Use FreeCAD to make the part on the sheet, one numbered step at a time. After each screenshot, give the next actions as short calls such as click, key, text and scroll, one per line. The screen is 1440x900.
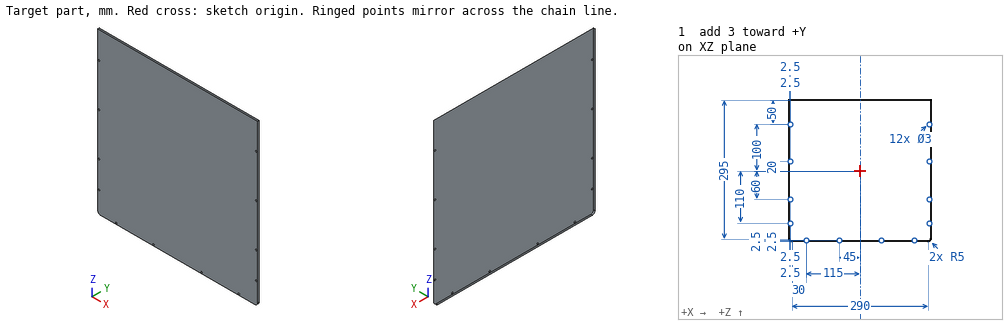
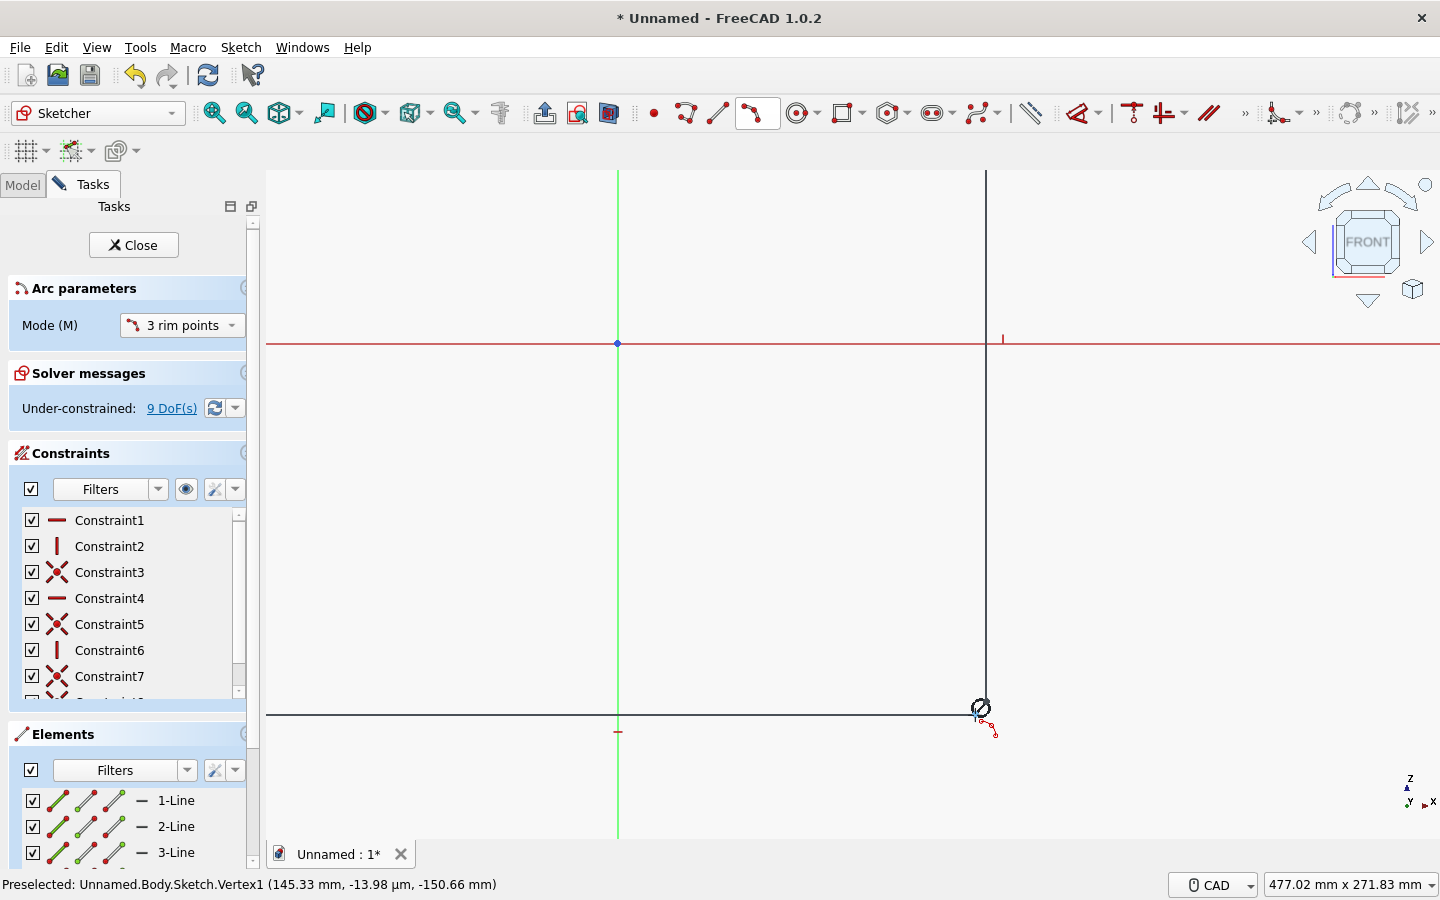
scroll(983, 709, up, 8)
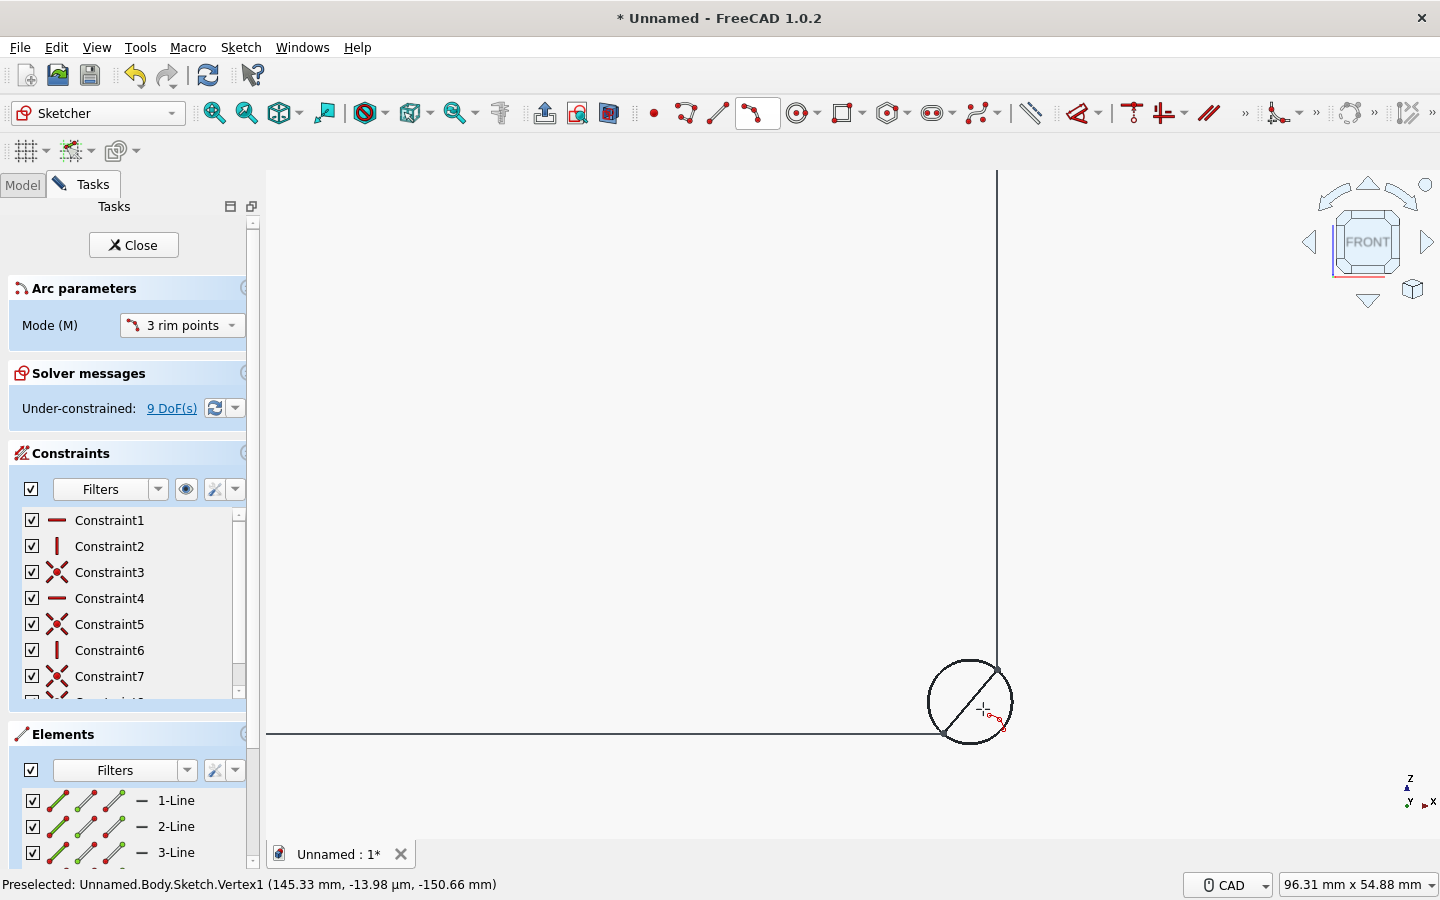
click(982, 708)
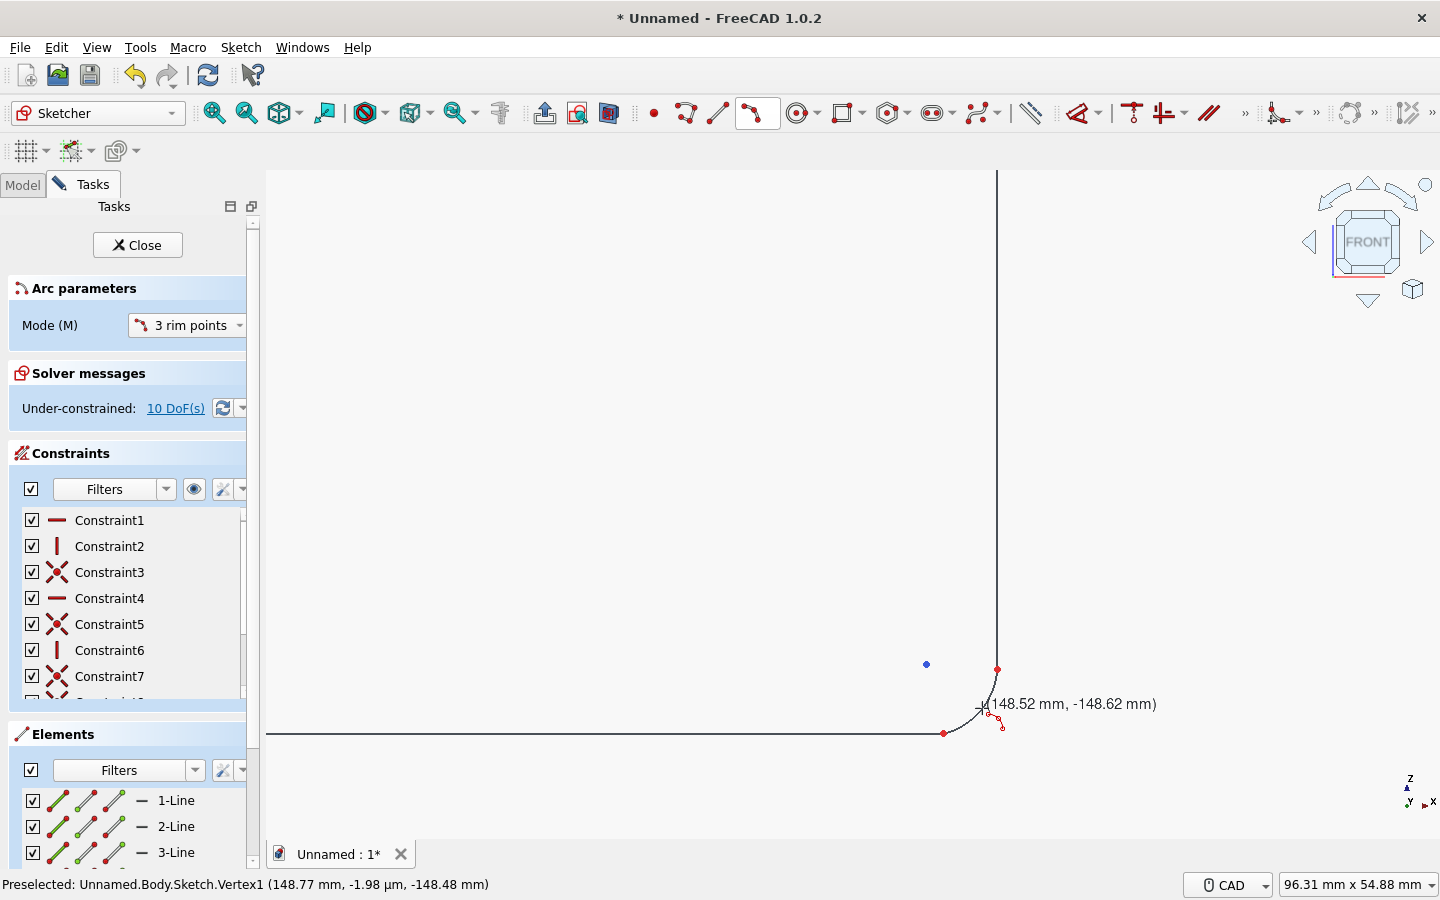
click(798, 114)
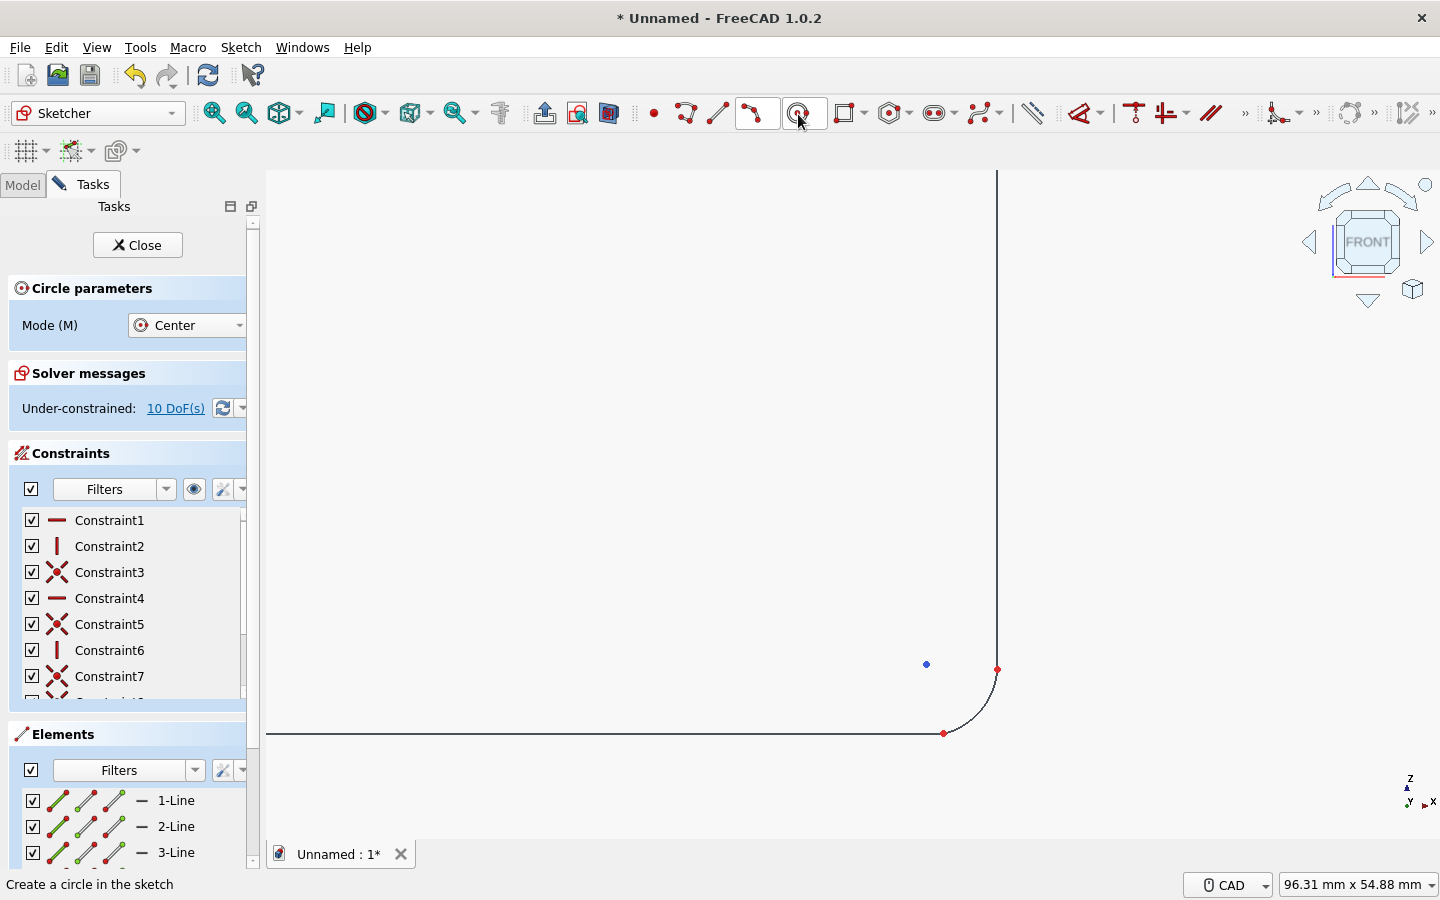
scroll(985, 705, down, 11)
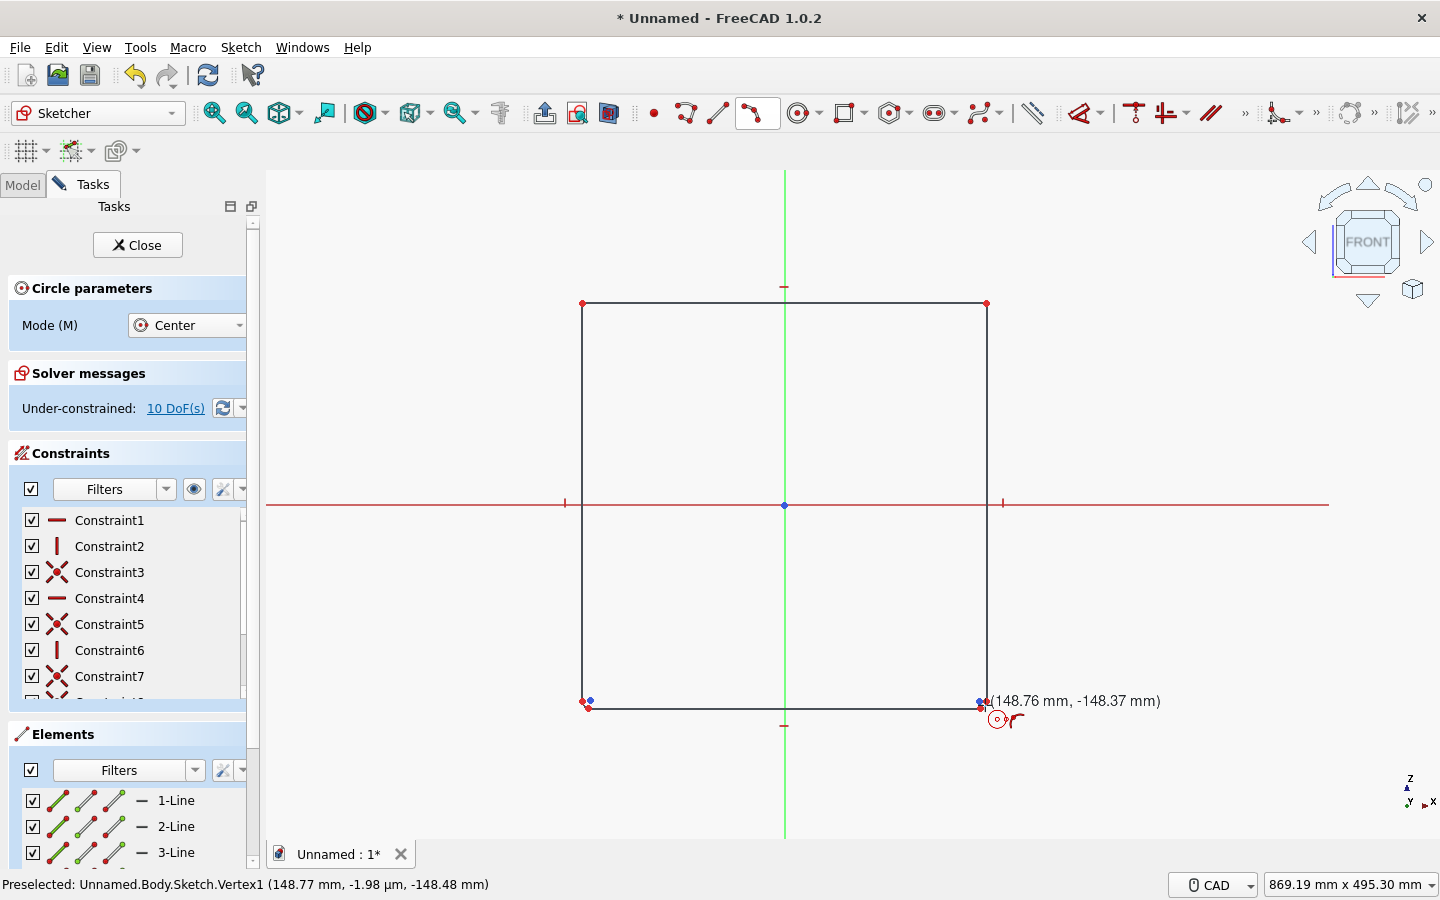
scroll(585, 370, up, 13)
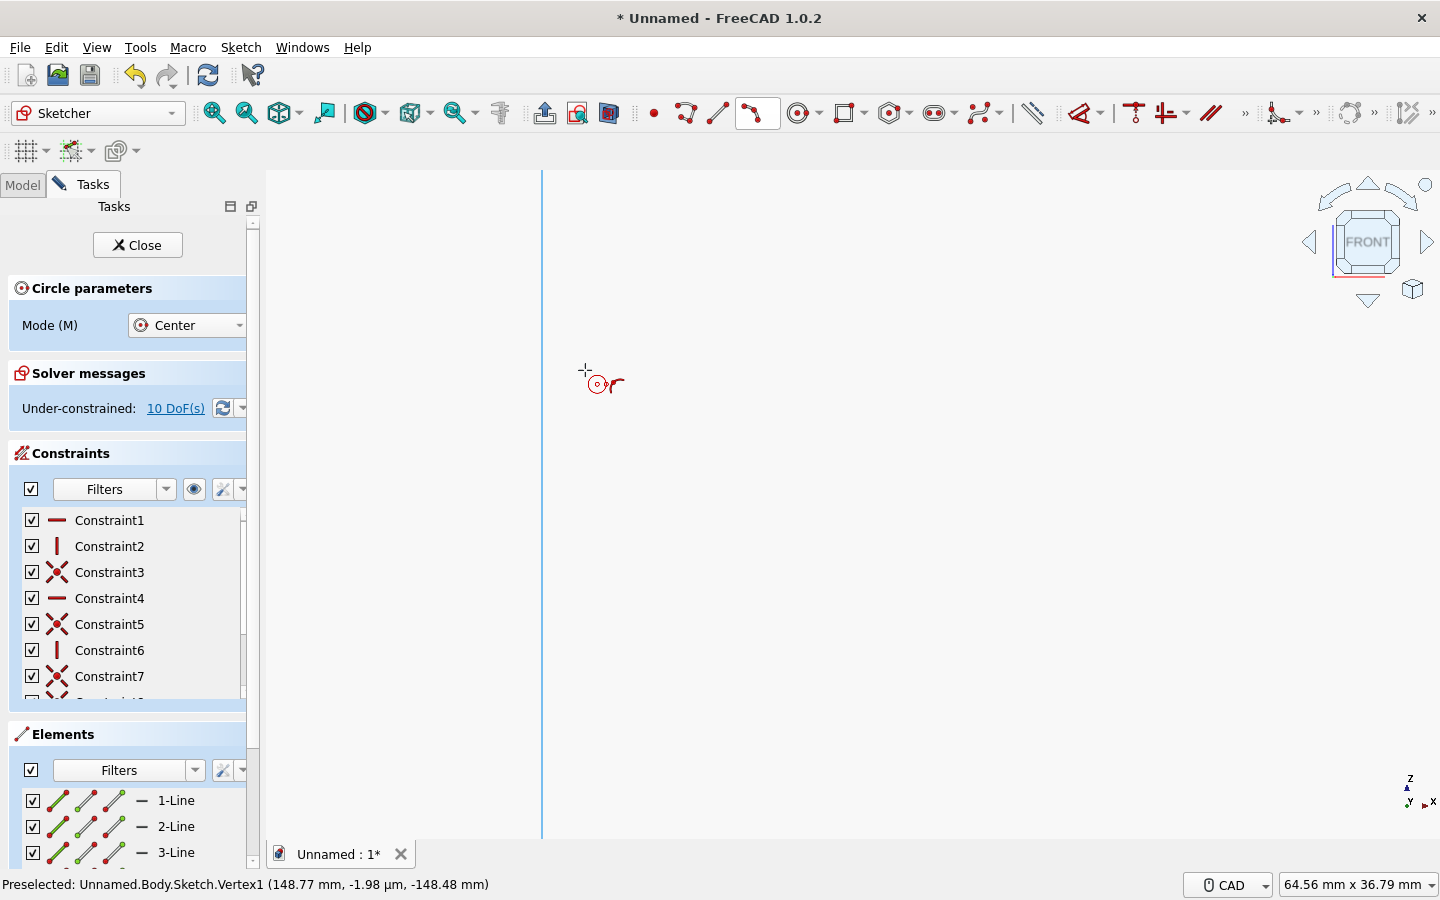
click(587, 371)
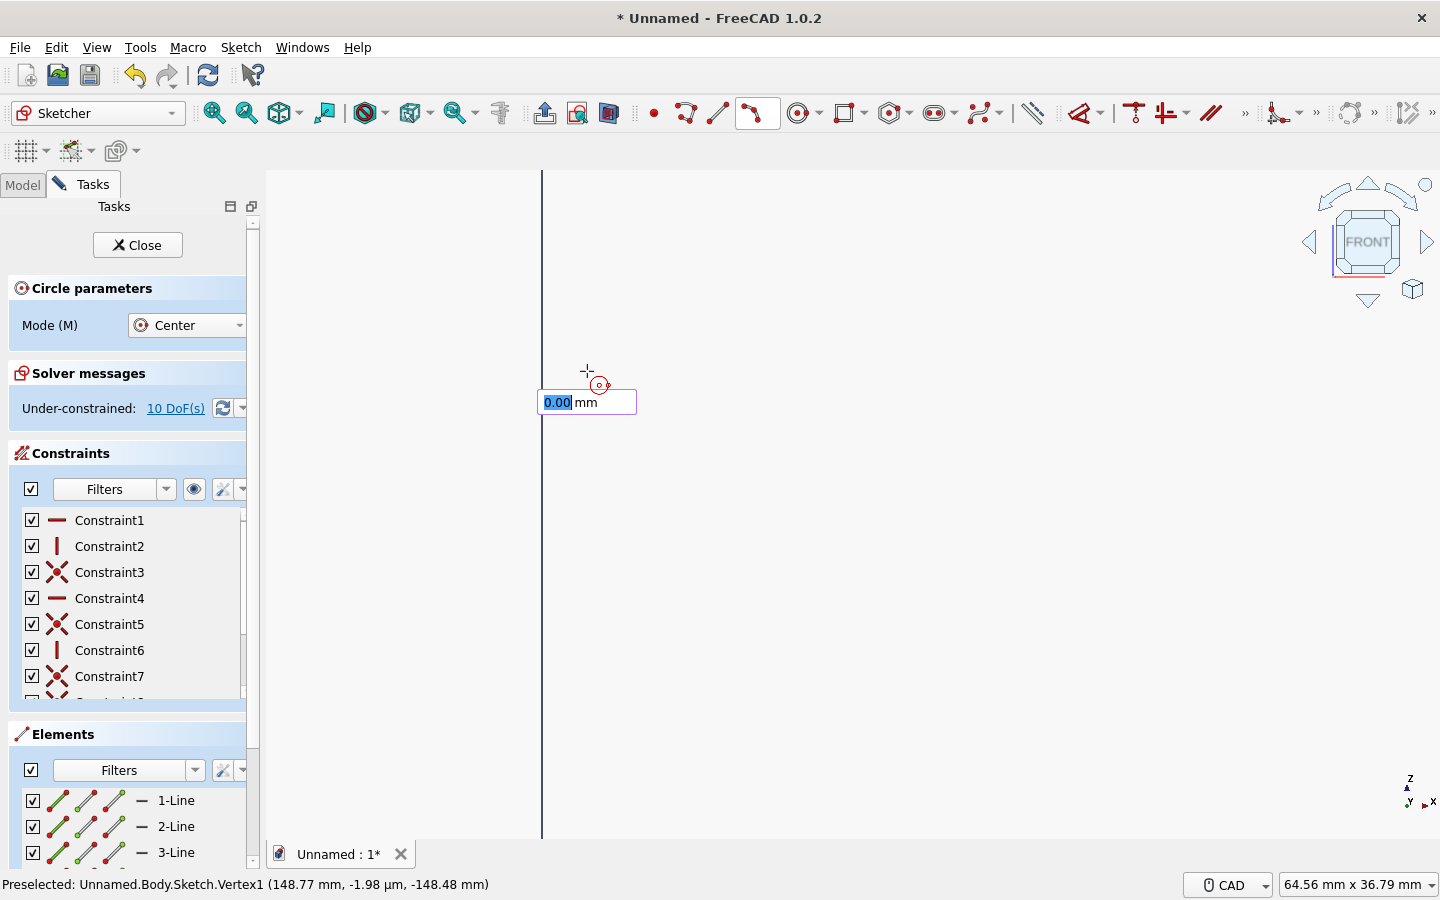
scroll(585, 369, down, 13)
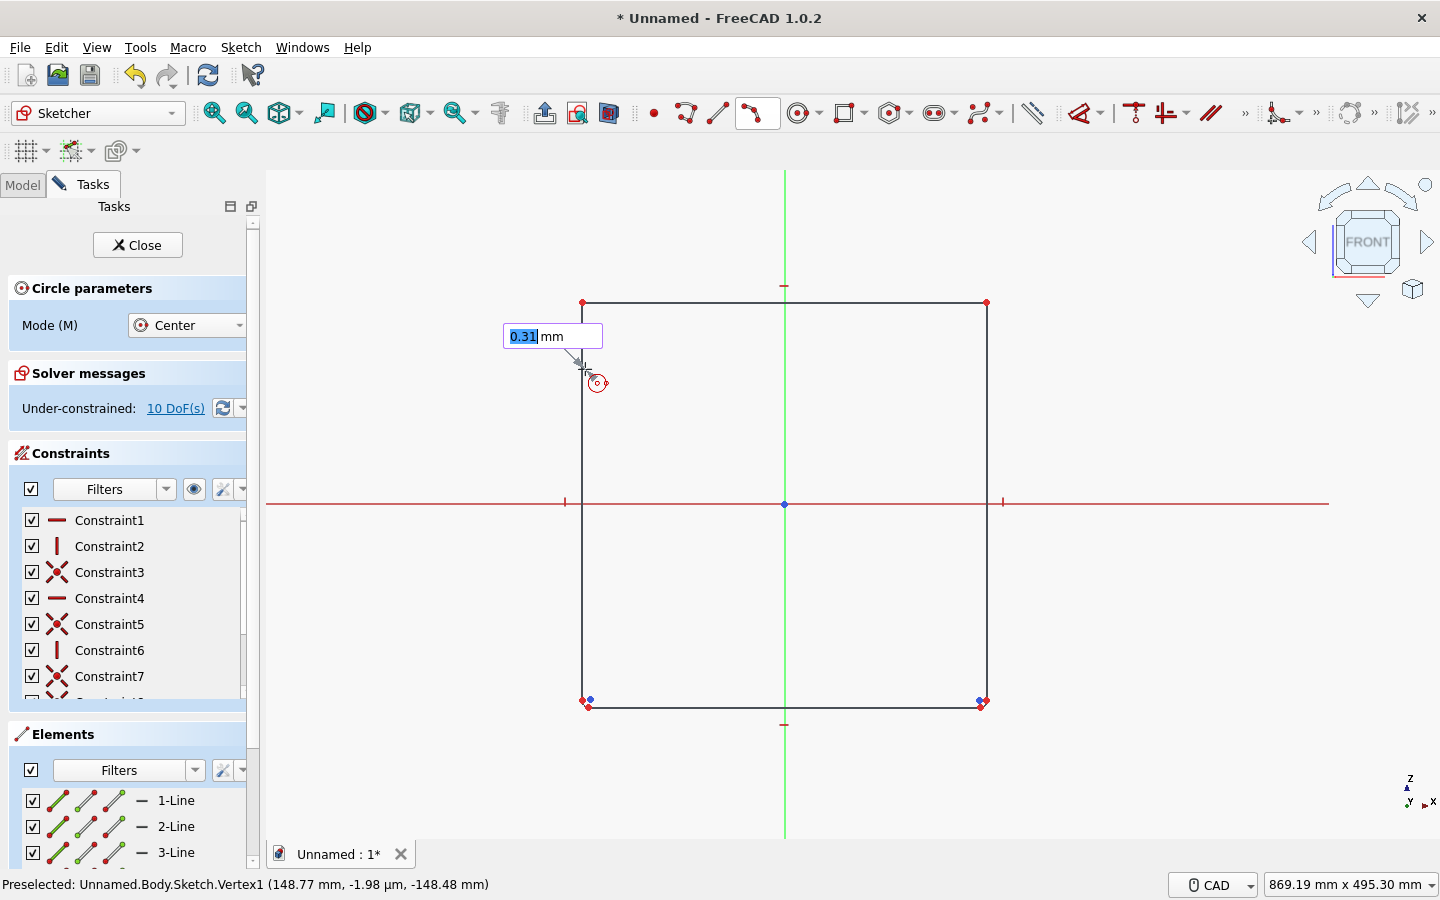
scroll(587, 368, up, 6)
move(586, 367)